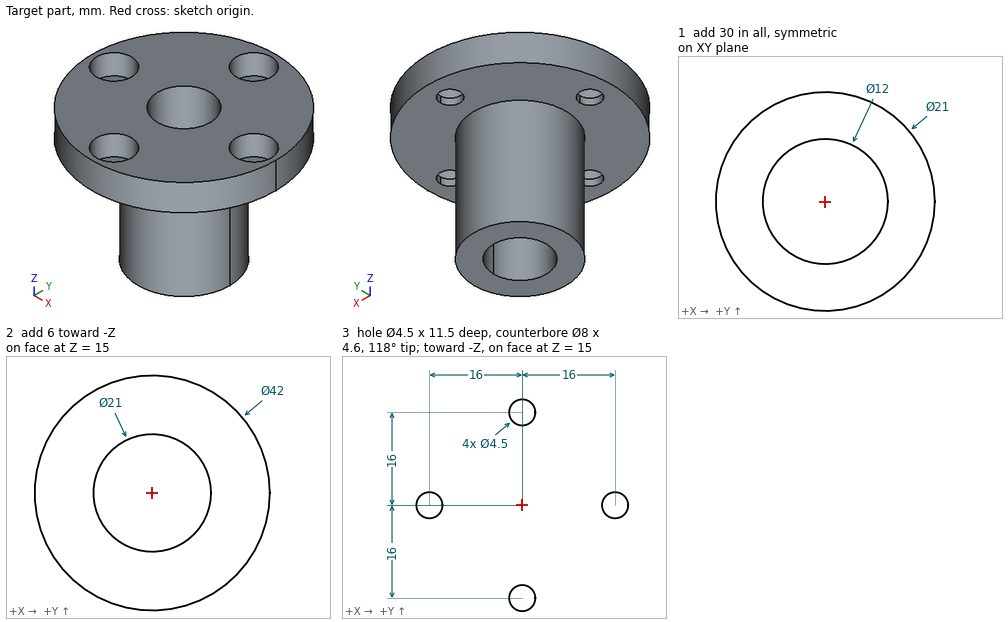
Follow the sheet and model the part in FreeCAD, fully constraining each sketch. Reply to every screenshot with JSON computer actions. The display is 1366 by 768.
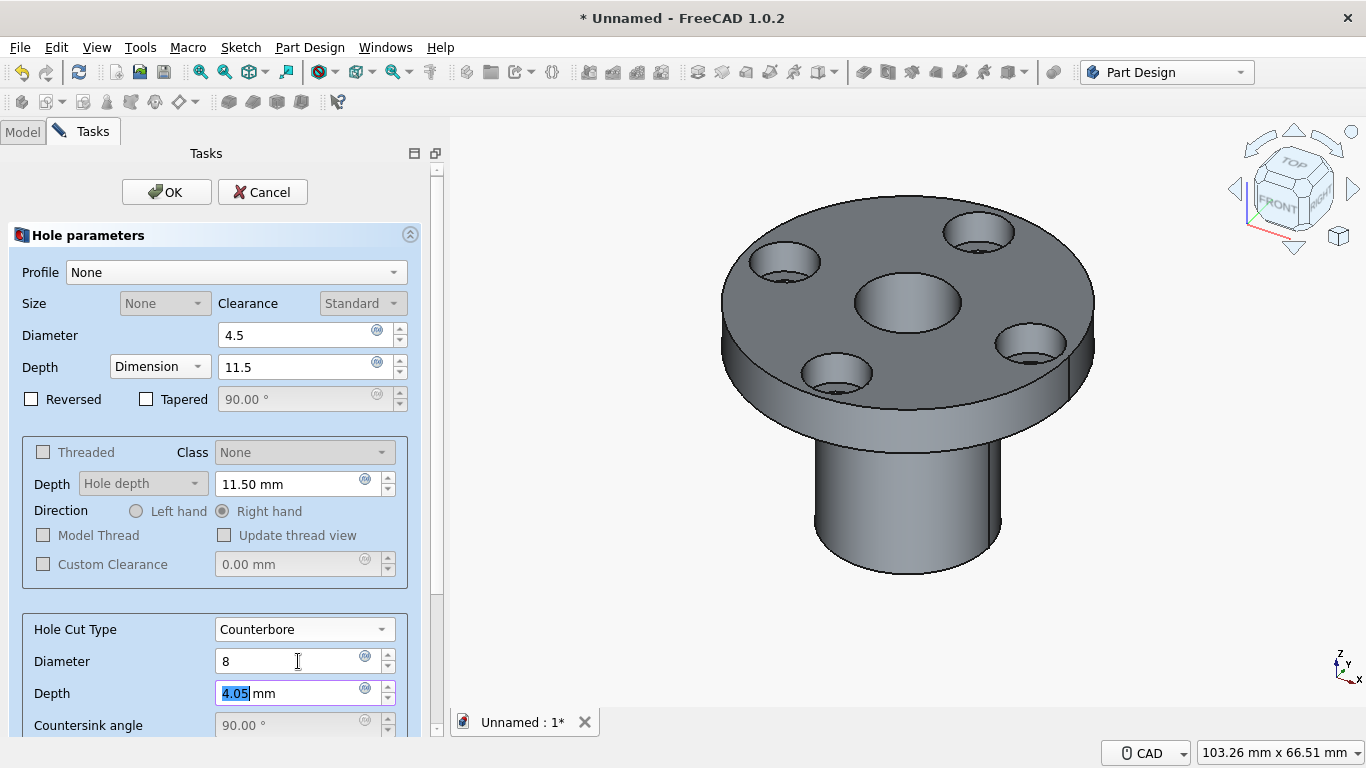
{"action": "type", "text": "4.6"}
{"action": "key", "text": "Tab"}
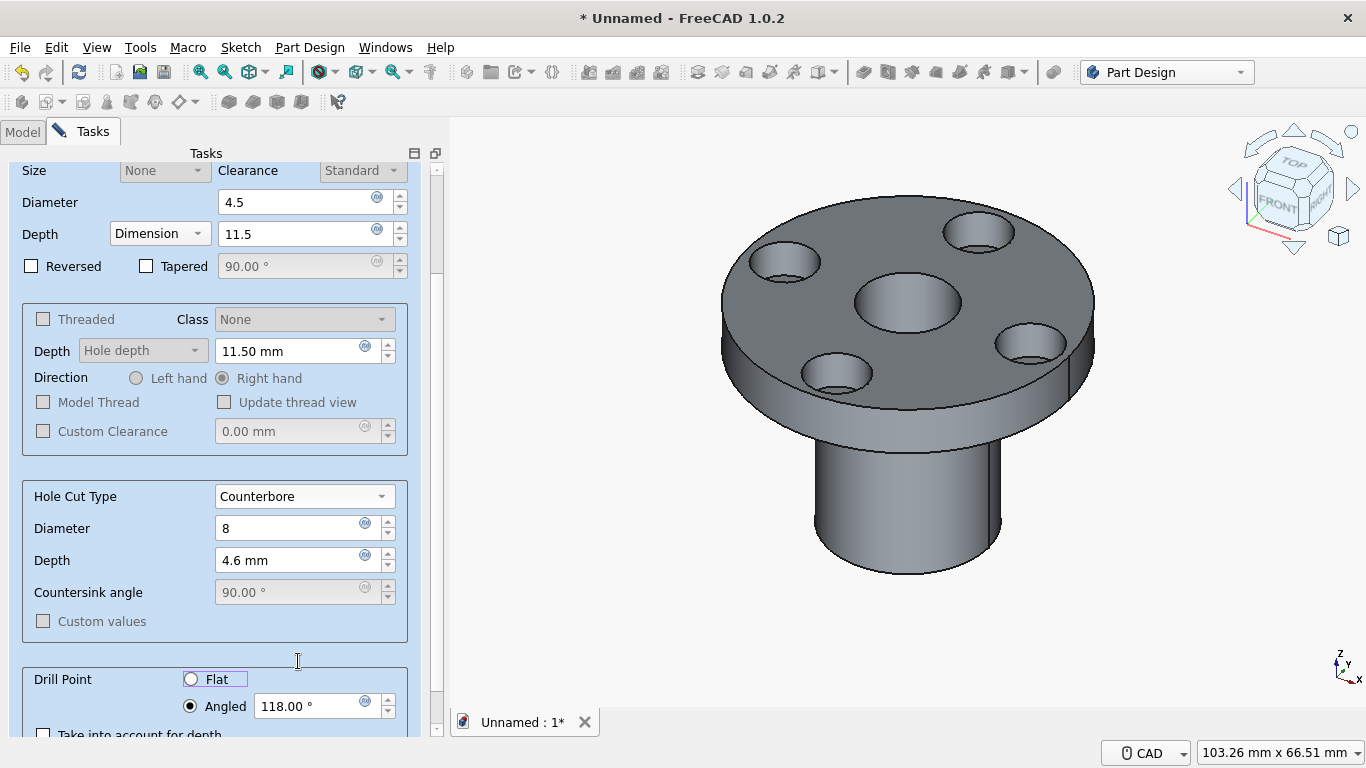
{"action": "scroll", "coordinate": [437, 450], "scroll_direction": "up", "scroll_amount": 3}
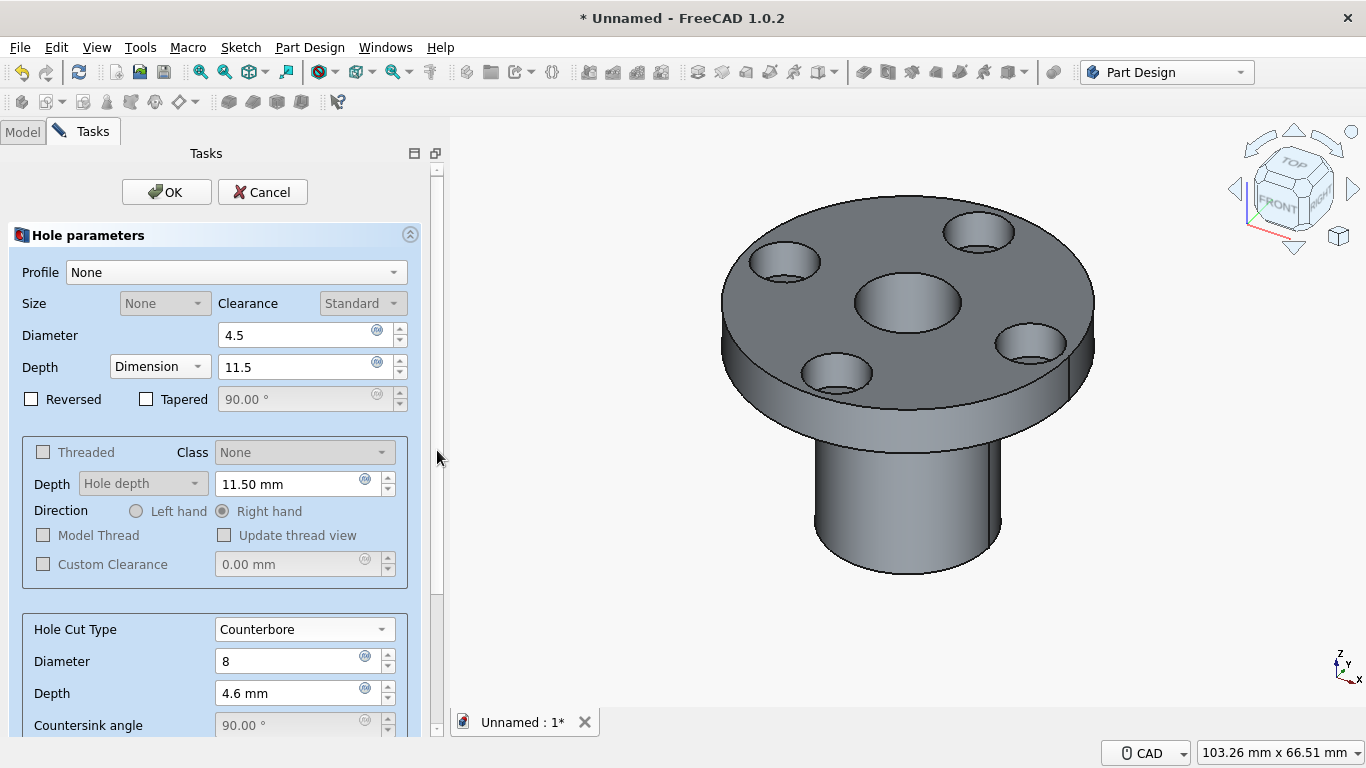
{"action": "left_click", "coordinate": [167, 192]}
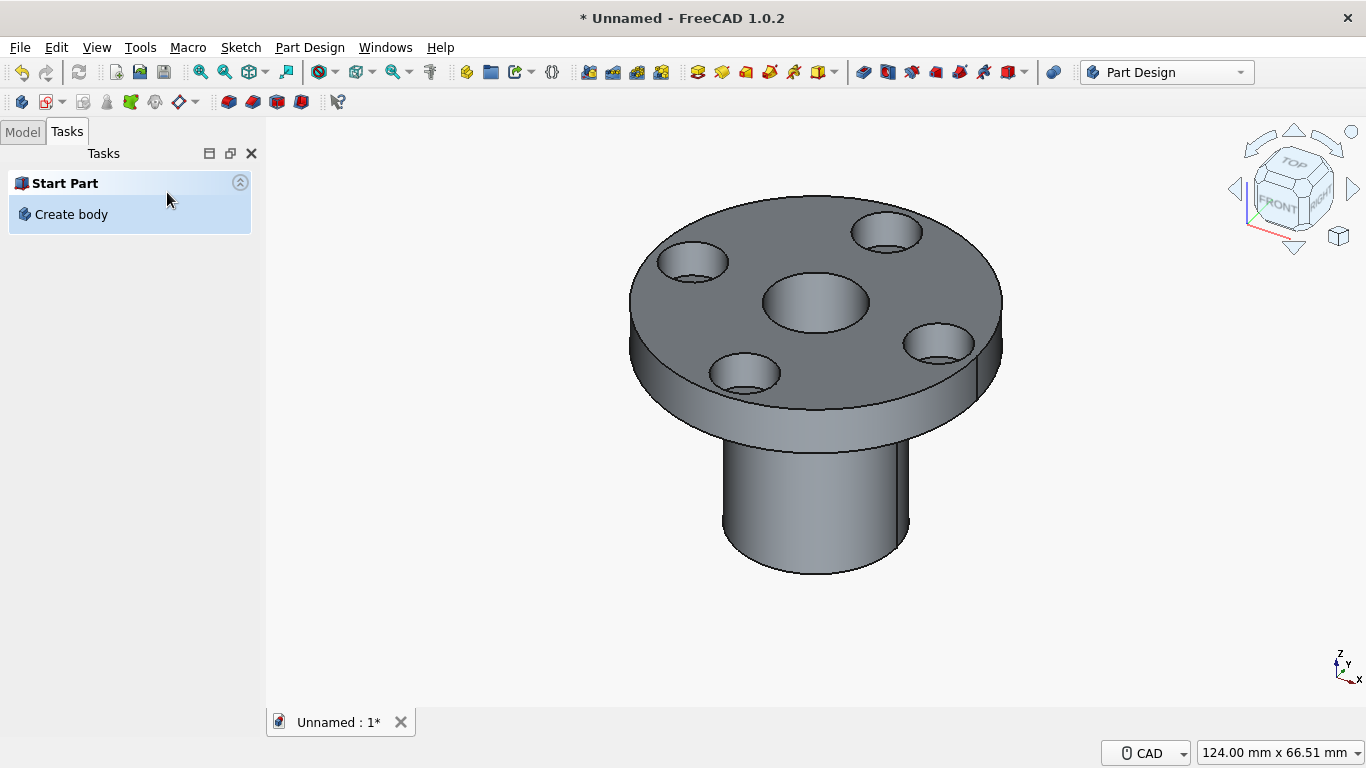
{"action": "key", "text": "0"}